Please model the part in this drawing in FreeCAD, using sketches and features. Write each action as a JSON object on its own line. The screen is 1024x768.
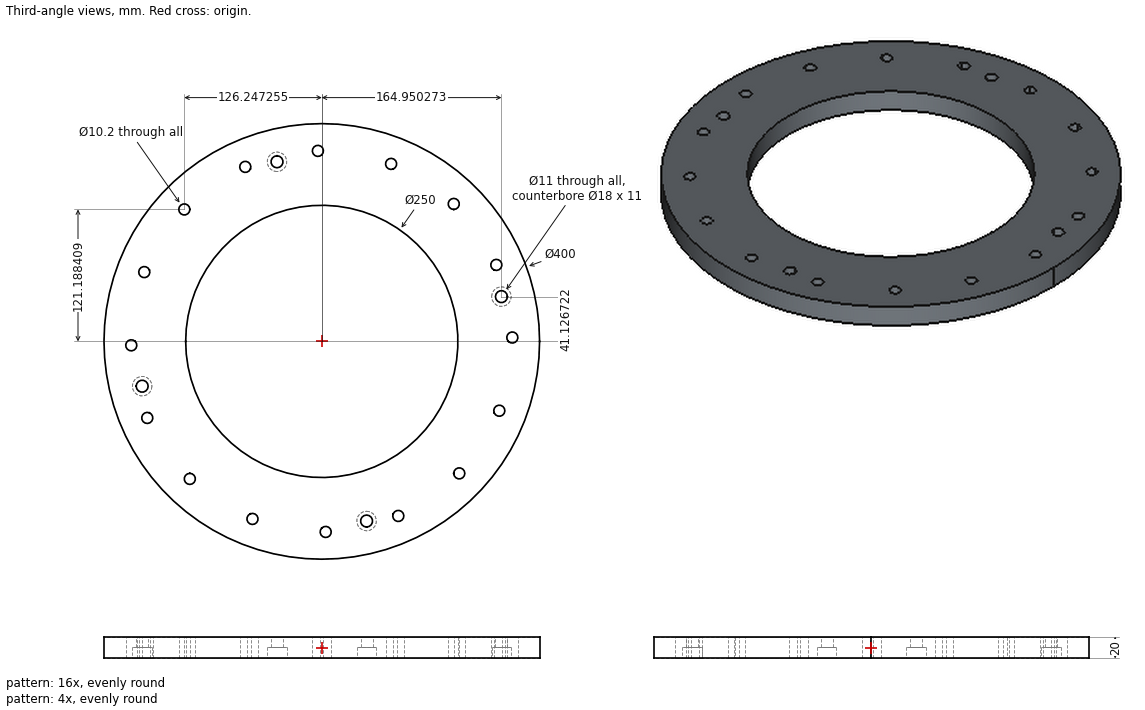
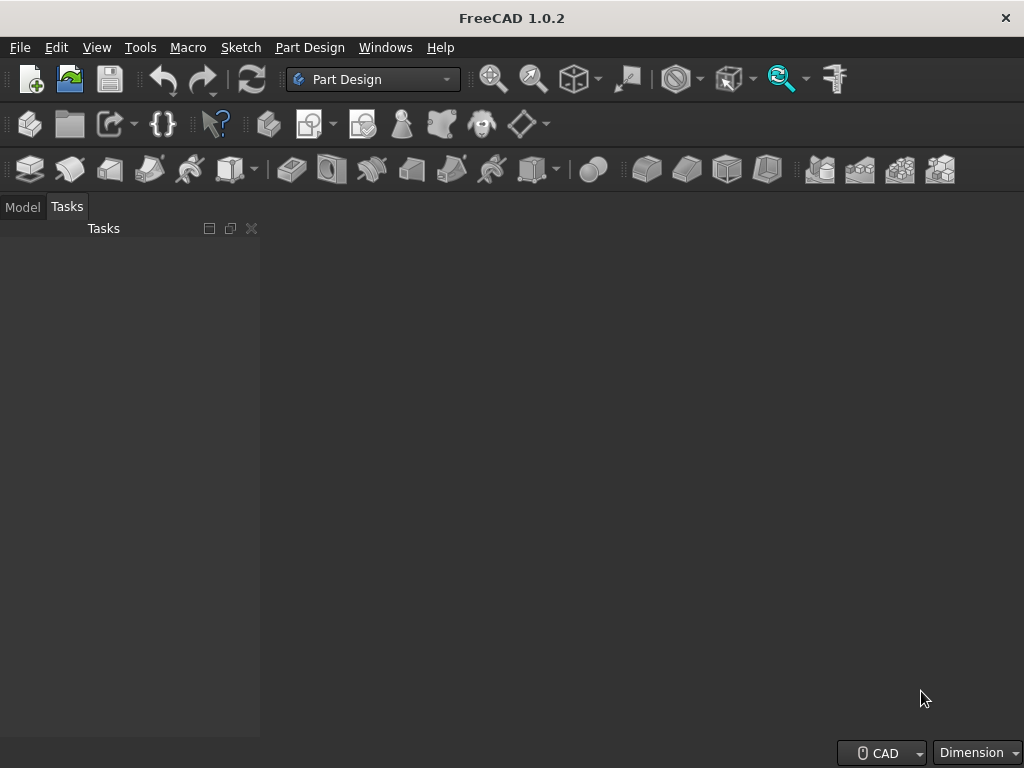
{"action": "key", "text": "ctrl+n"}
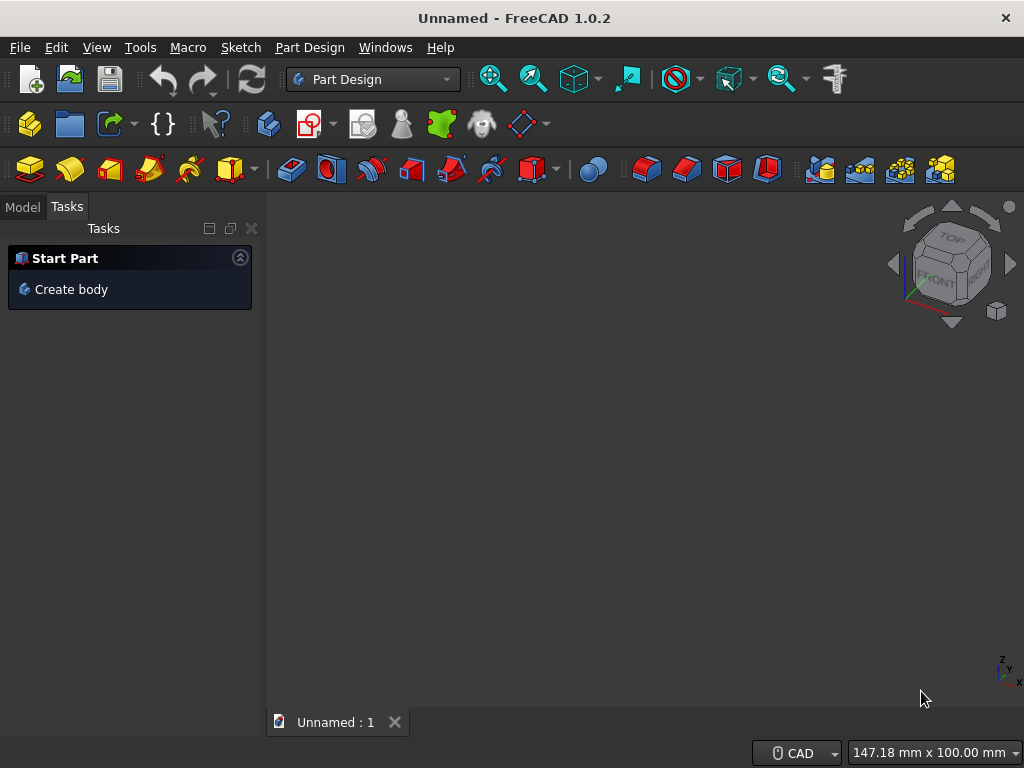
{"action": "left_click", "coordinate": [310, 124]}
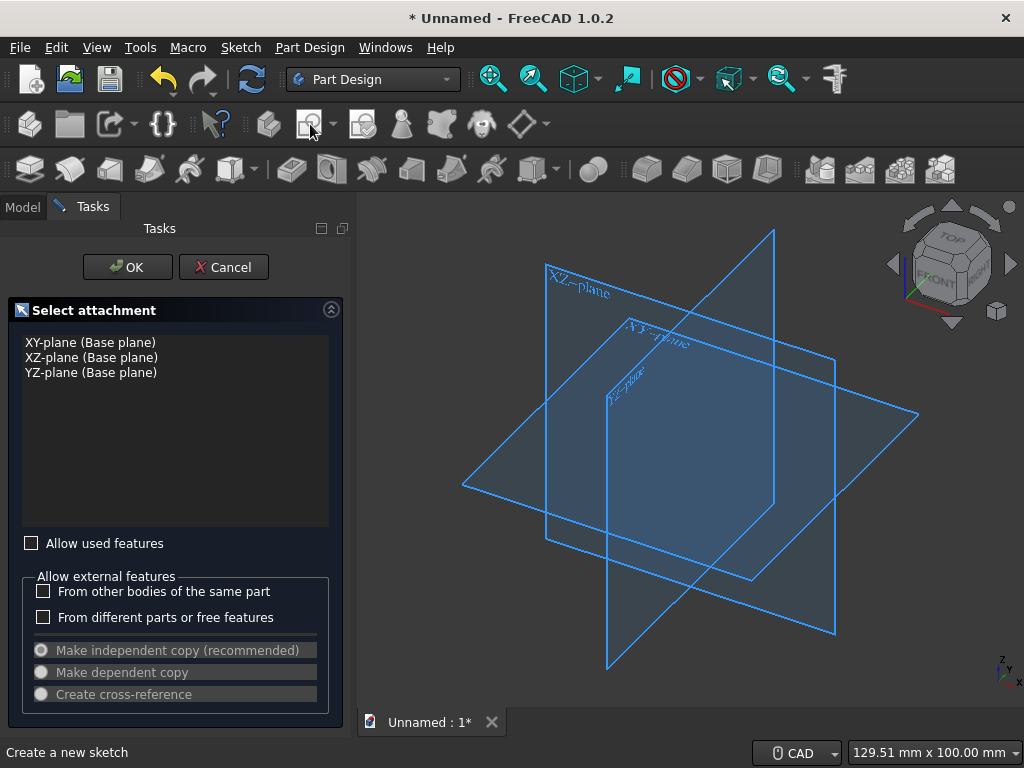
{"action": "left_click", "coordinate": [82, 342]}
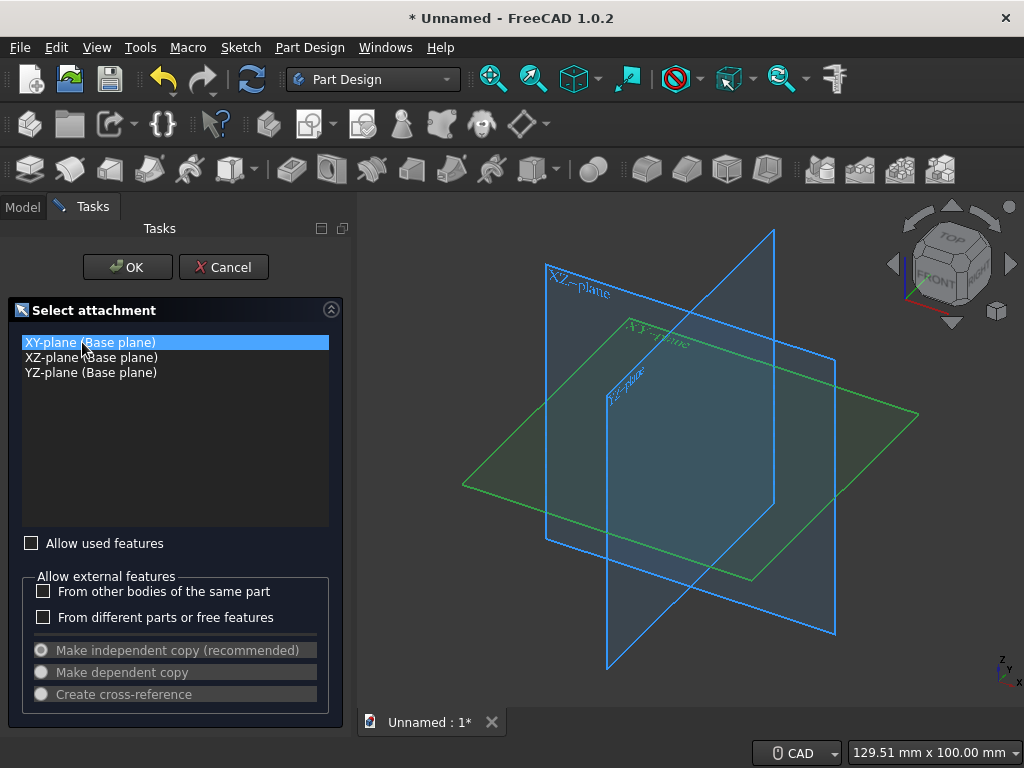
{"action": "left_click", "coordinate": [128, 267]}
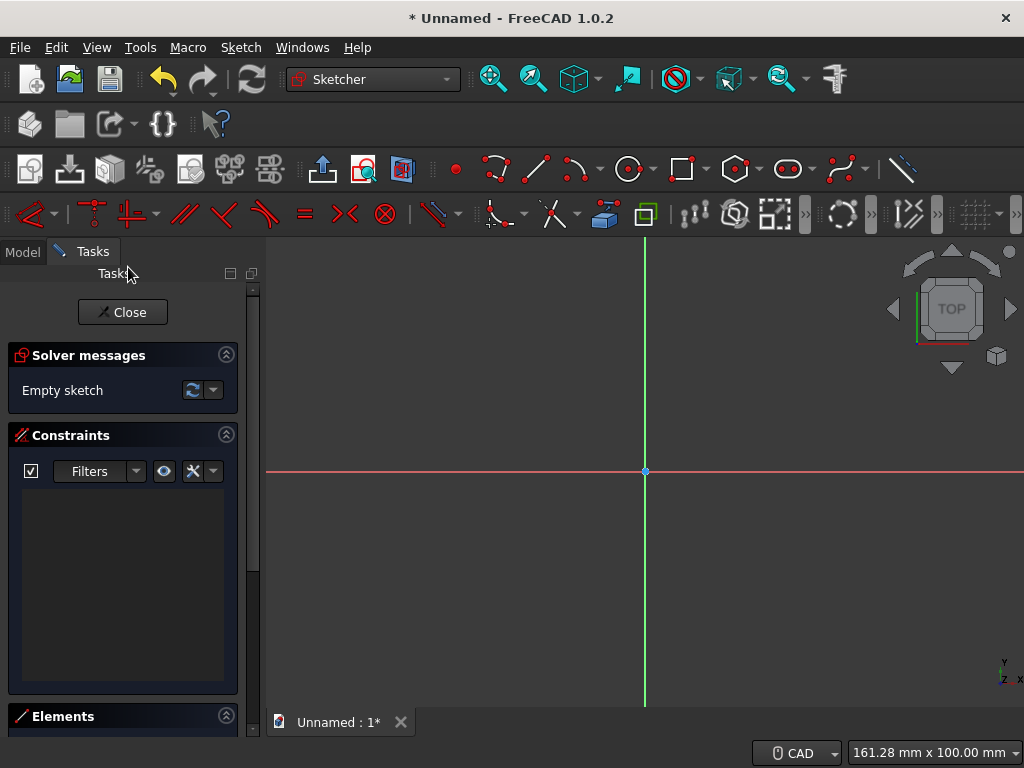
{"action": "scroll", "coordinate": [563, 472], "scroll_direction": "down", "scroll_amount": 9}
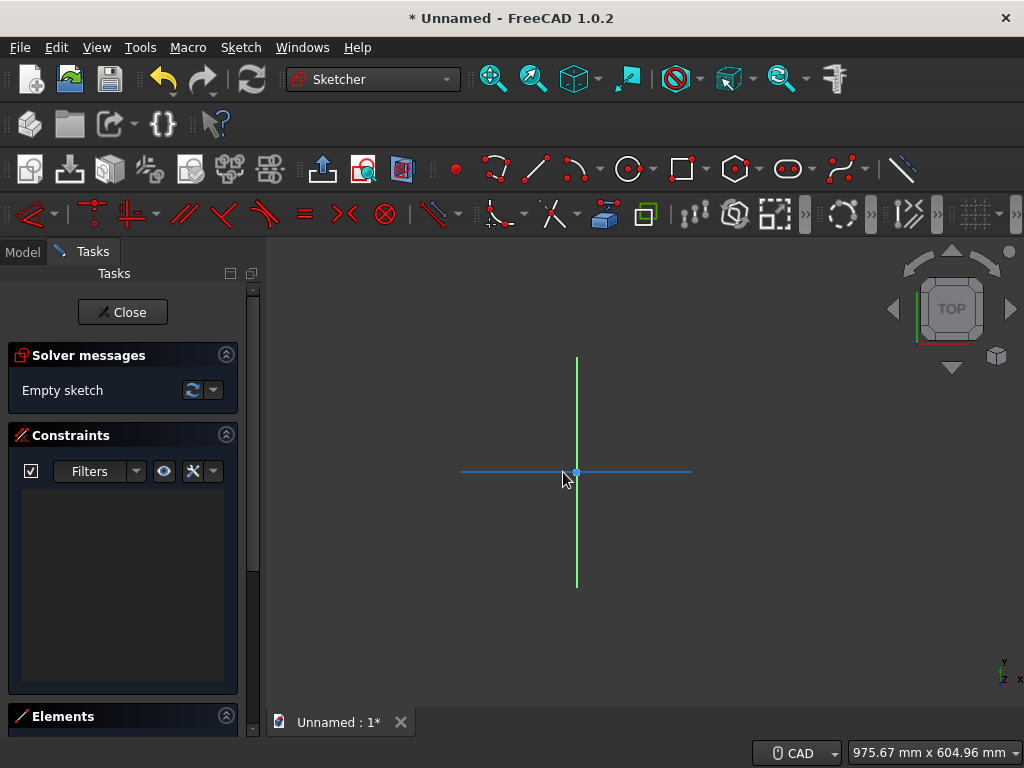
{"action": "key", "text": "g c"}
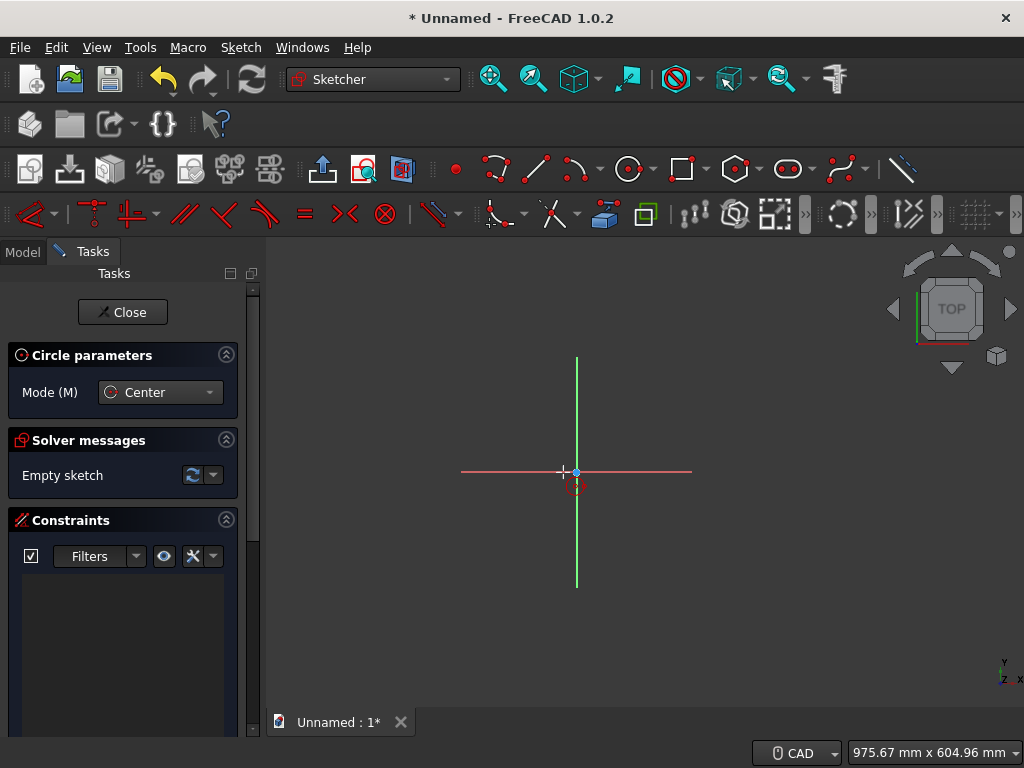
{"action": "left_click", "coordinate": [577, 472]}
{"action": "left_click", "coordinate": [687, 363]}
{"action": "key", "text": "Escape"}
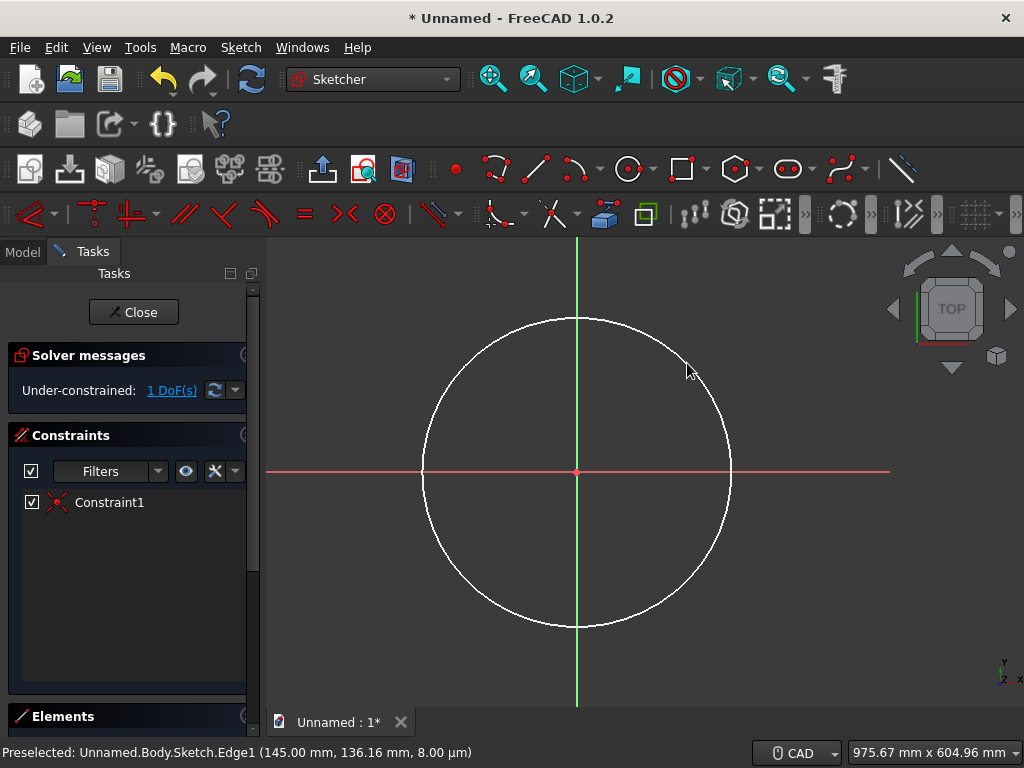
{"action": "left_click", "coordinate": [686, 363]}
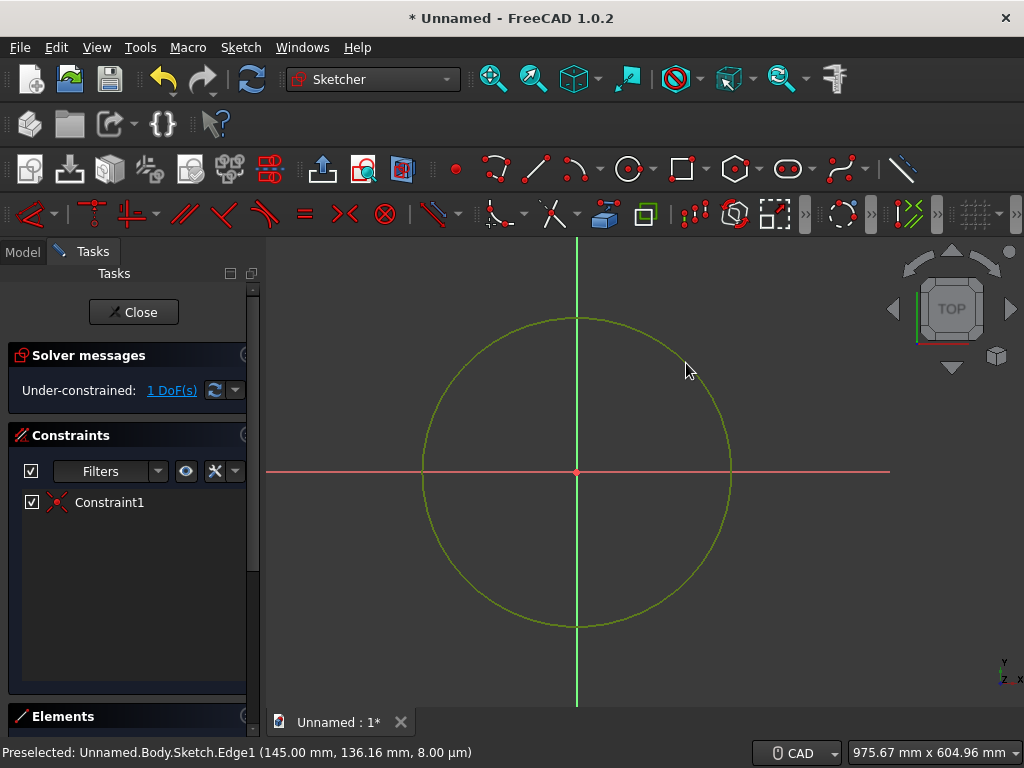
{"action": "left_click", "coordinate": [56, 214]}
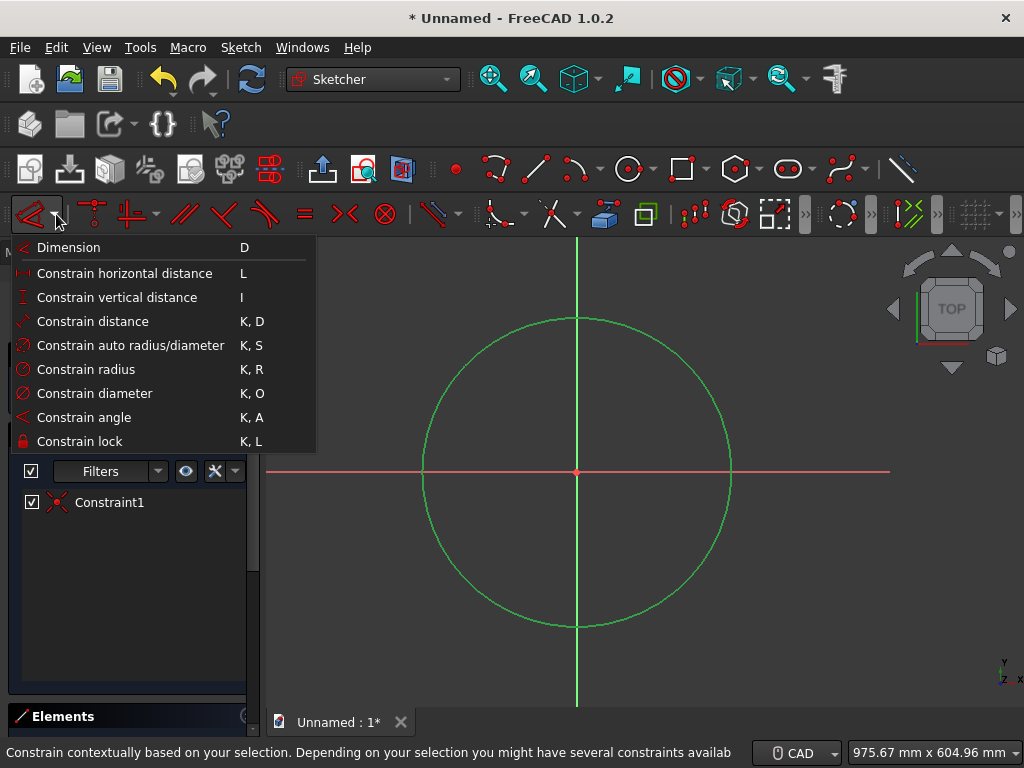
{"action": "left_click", "coordinate": [164, 393]}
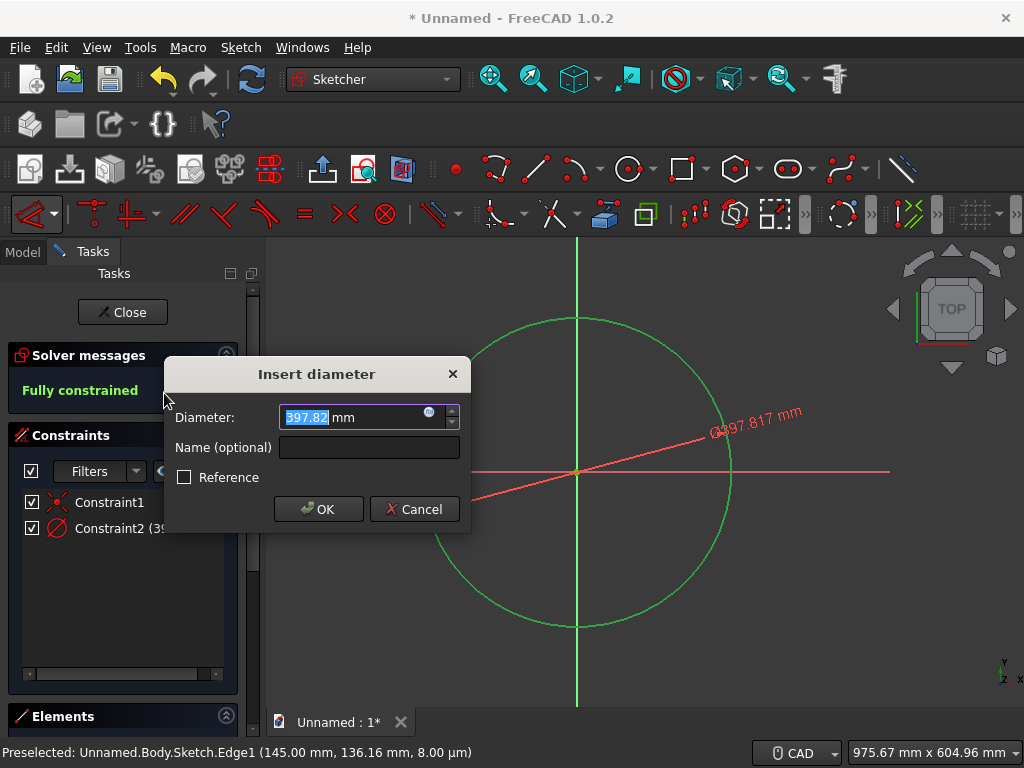
{"action": "type", "text": "400"}
{"action": "key", "text": "Return"}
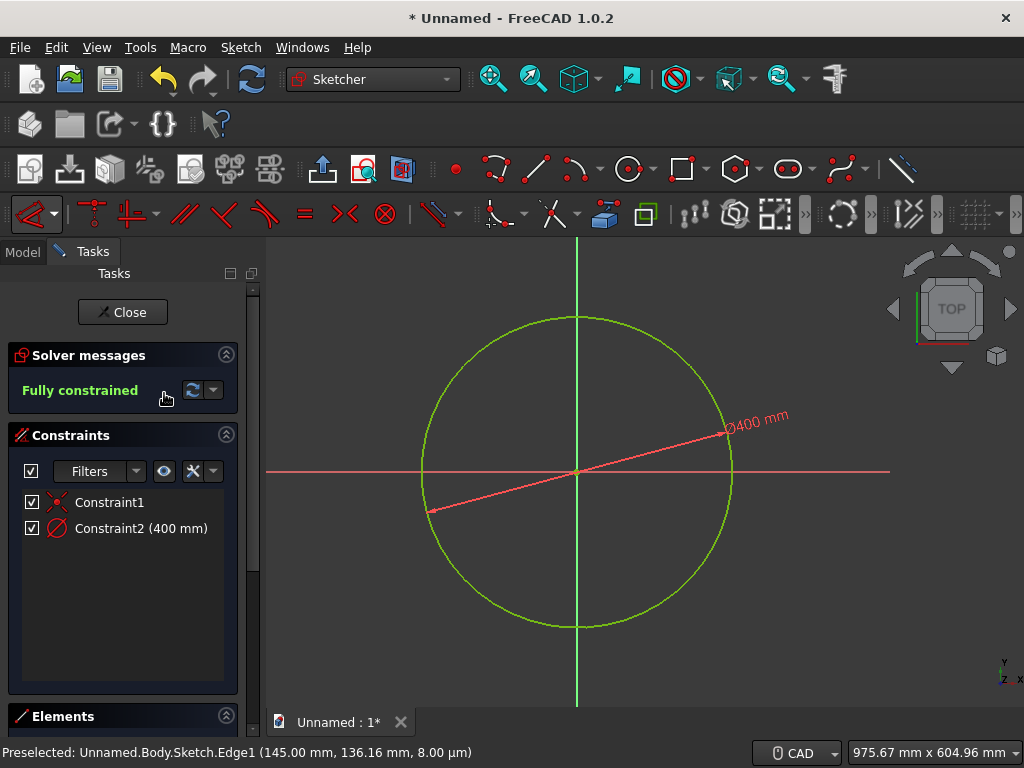
{"action": "left_click", "coordinate": [123, 312]}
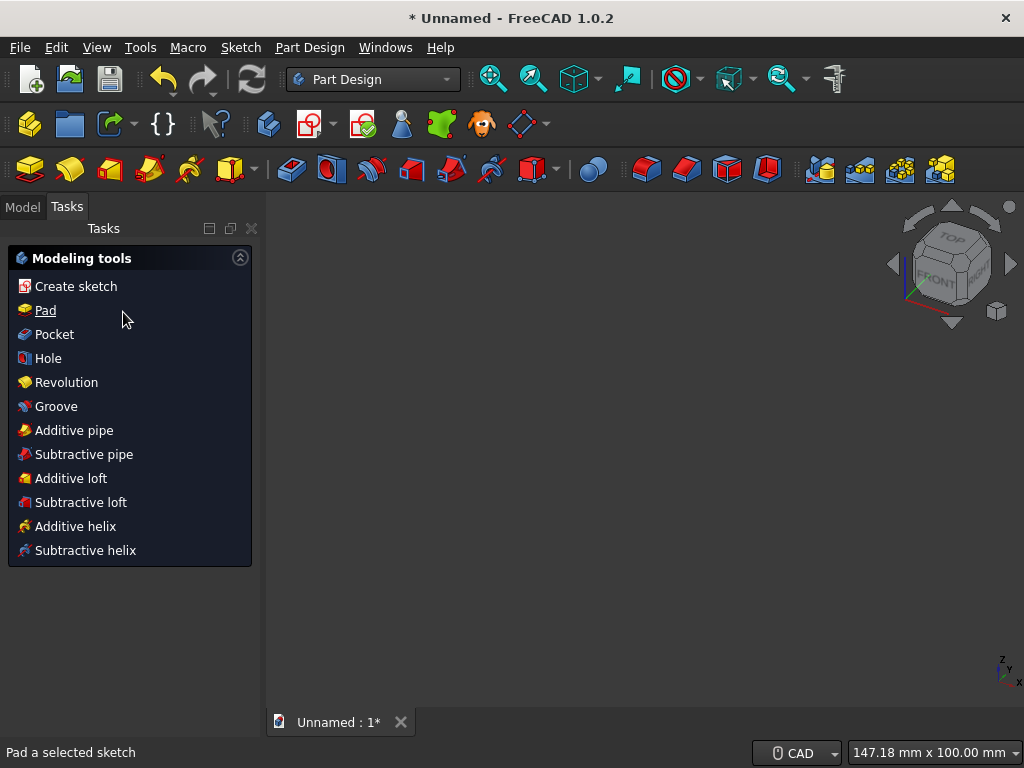
{"action": "left_click", "coordinate": [30, 170]}